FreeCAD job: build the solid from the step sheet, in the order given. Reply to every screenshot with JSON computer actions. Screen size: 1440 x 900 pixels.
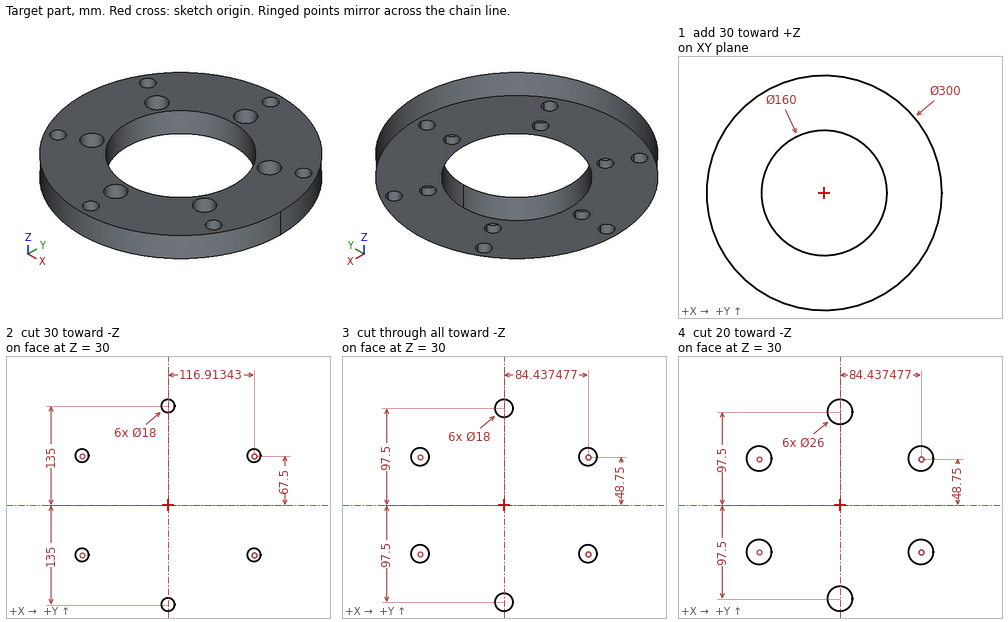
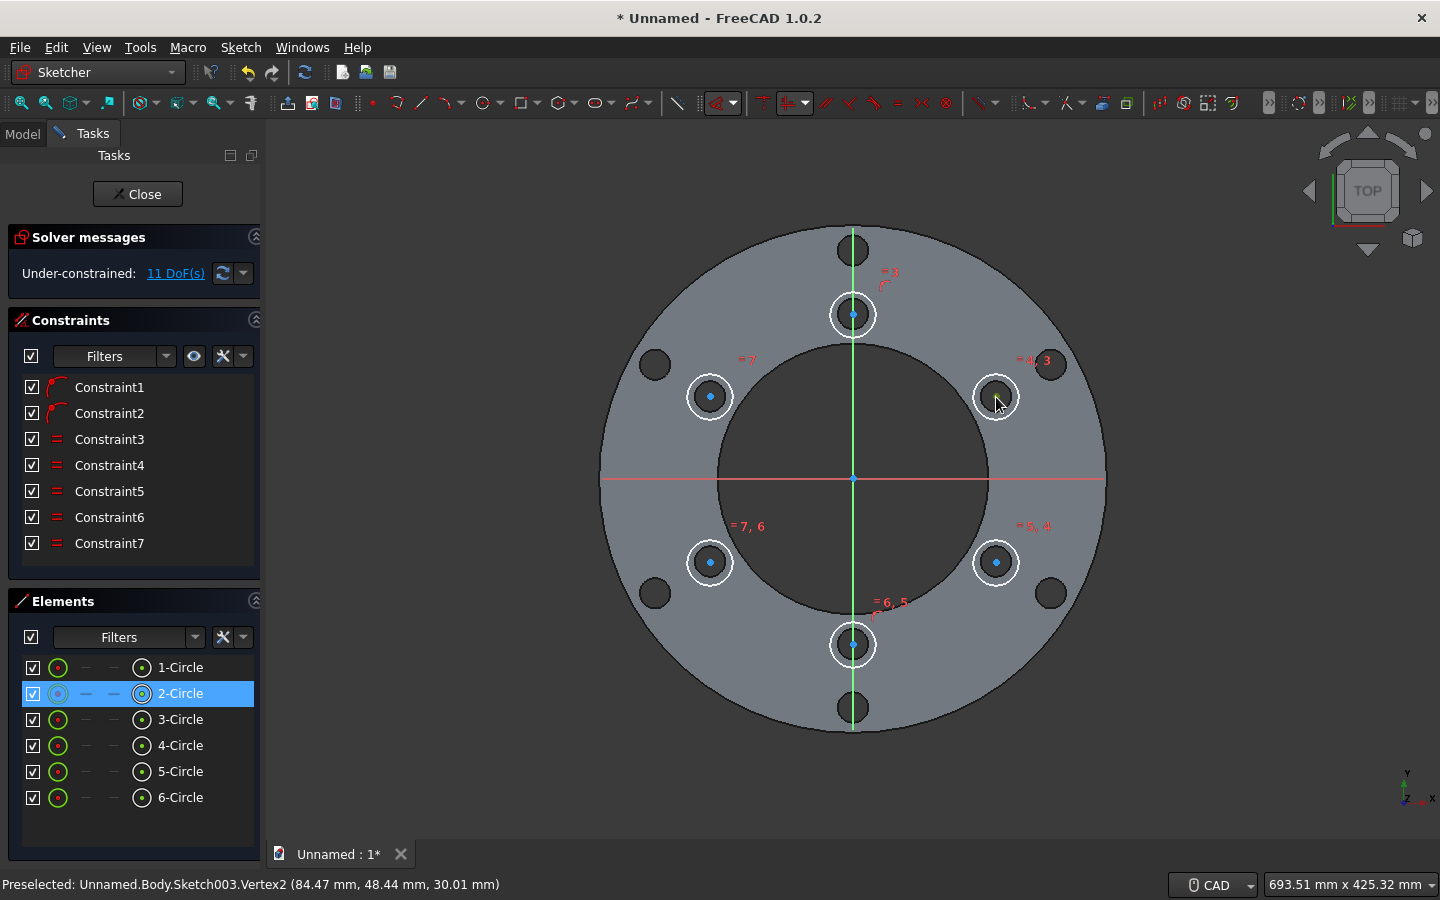
{"action": "left_click", "coordinate": [996, 563]}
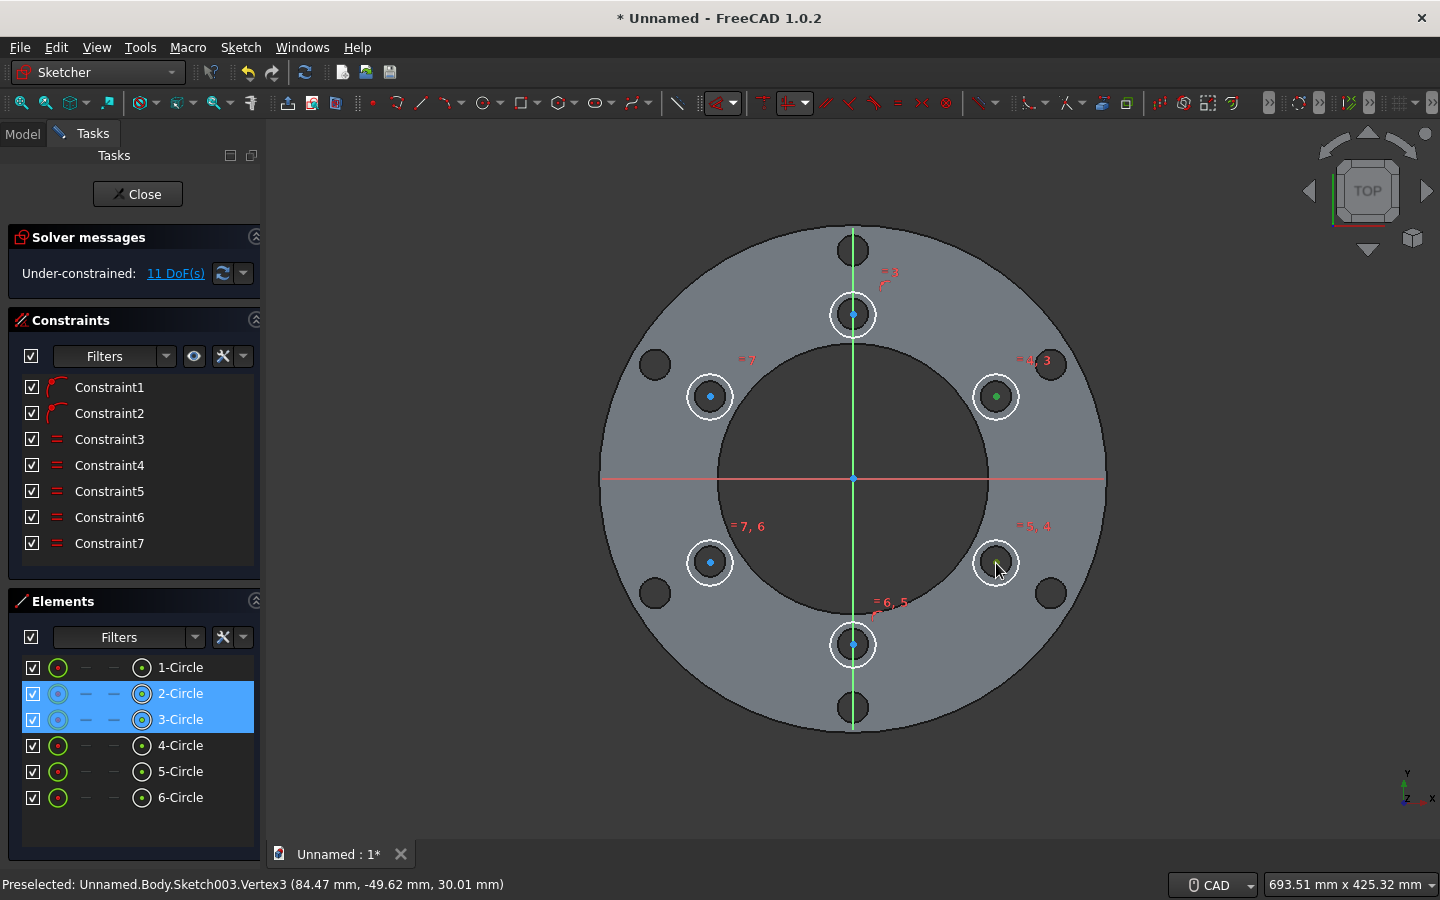
{"action": "left_click", "coordinate": [644, 479]}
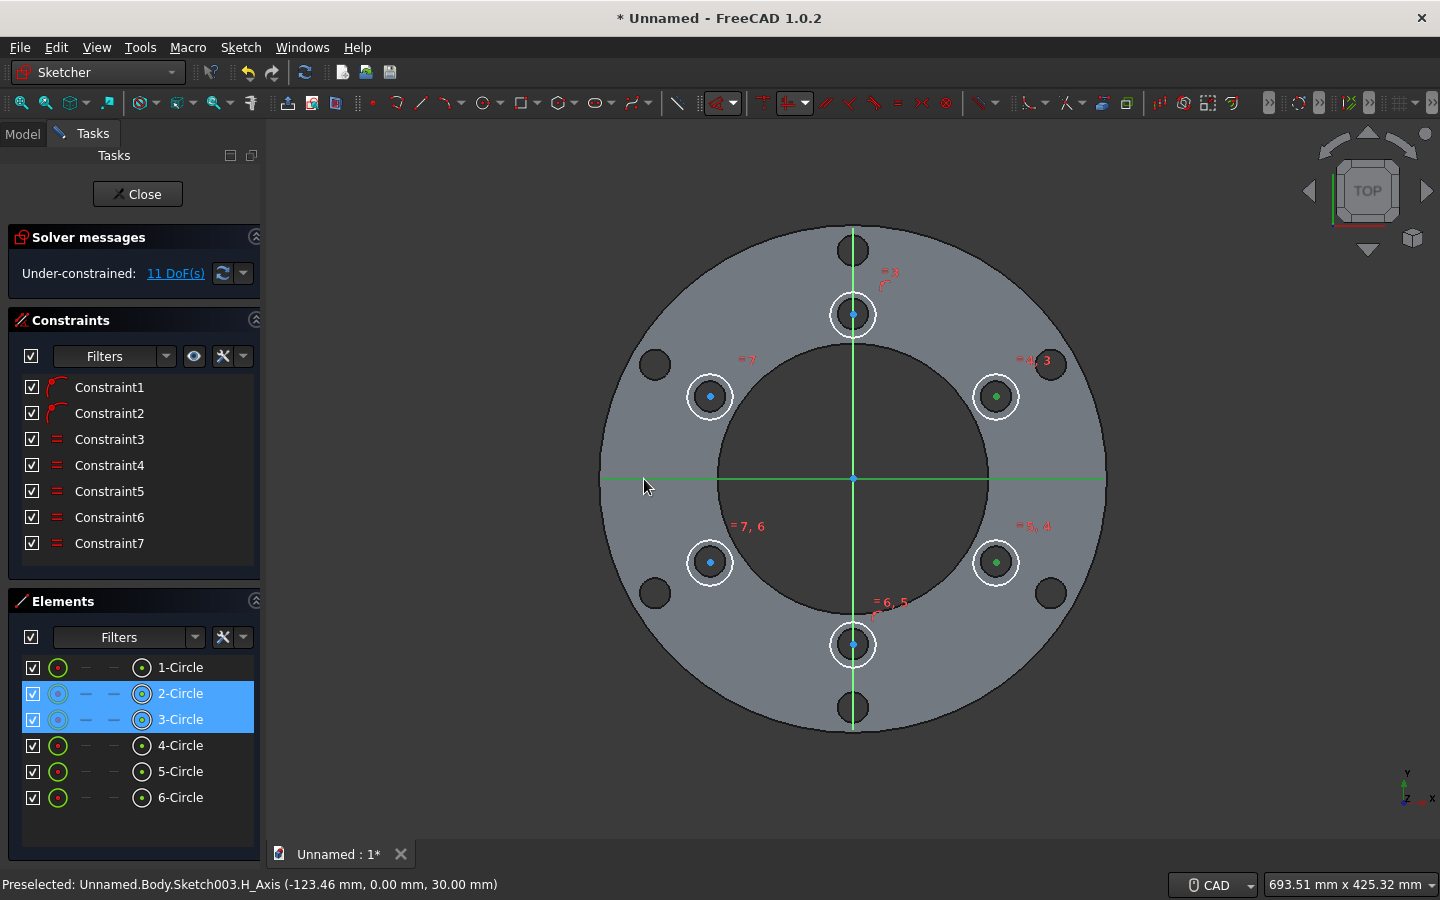
{"action": "left_click", "coordinate": [922, 104]}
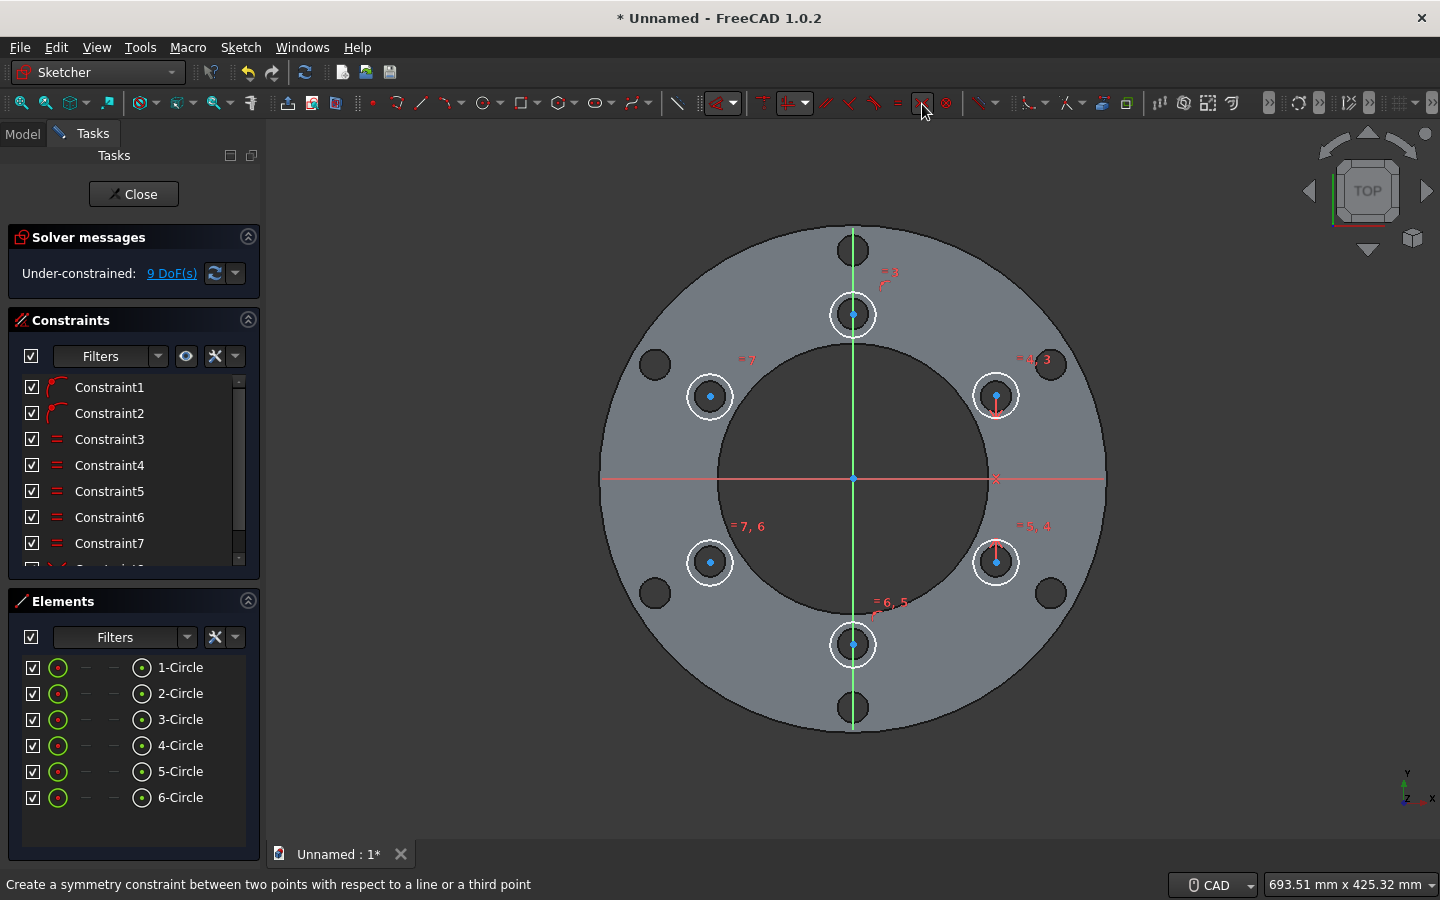
{"action": "left_click", "coordinate": [996, 563]}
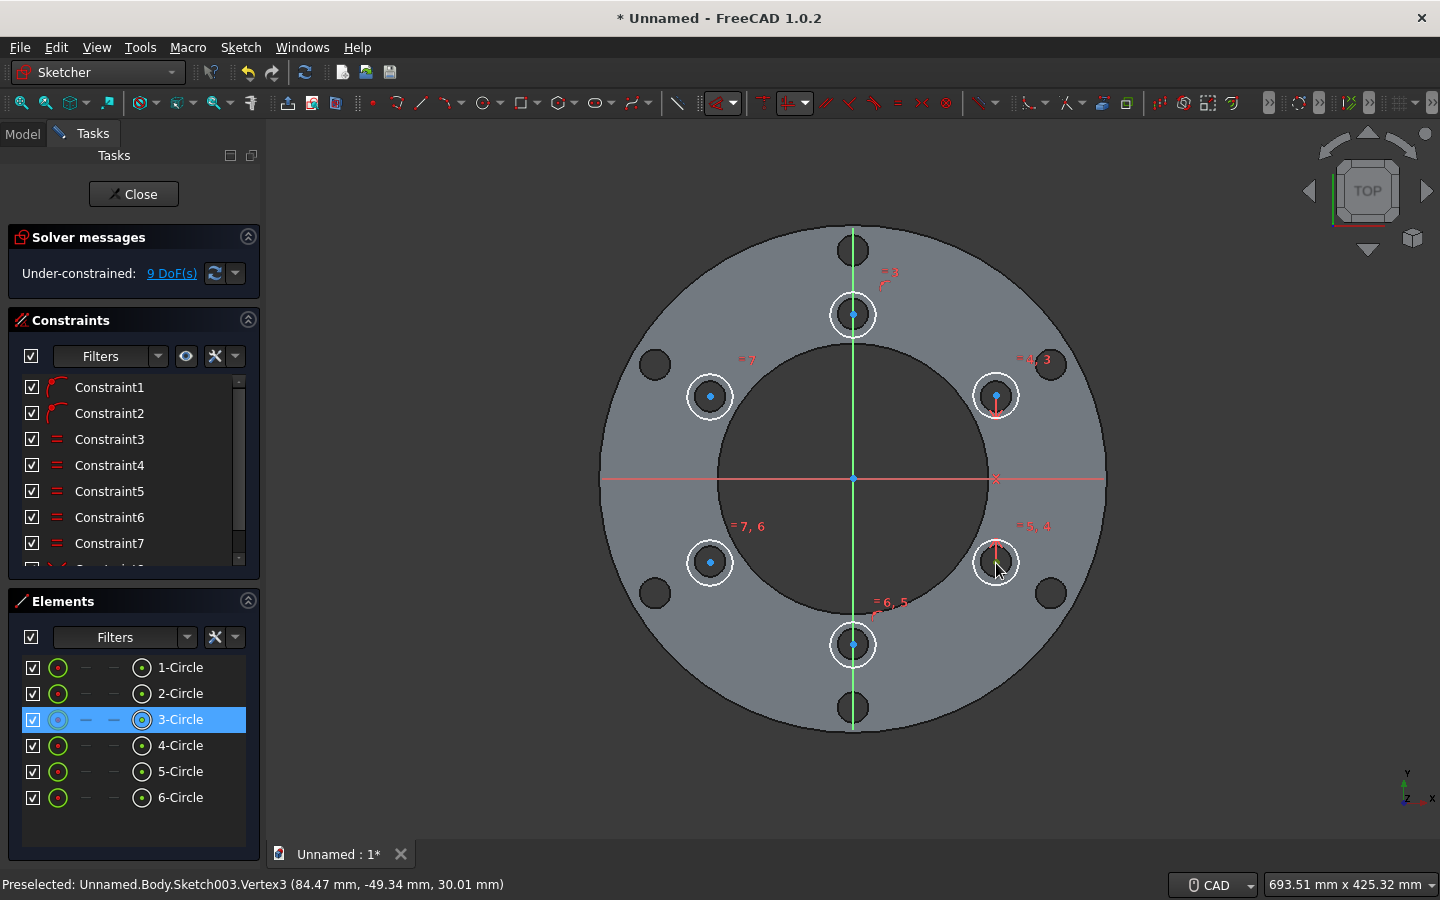
{"action": "left_click", "coordinate": [710, 563]}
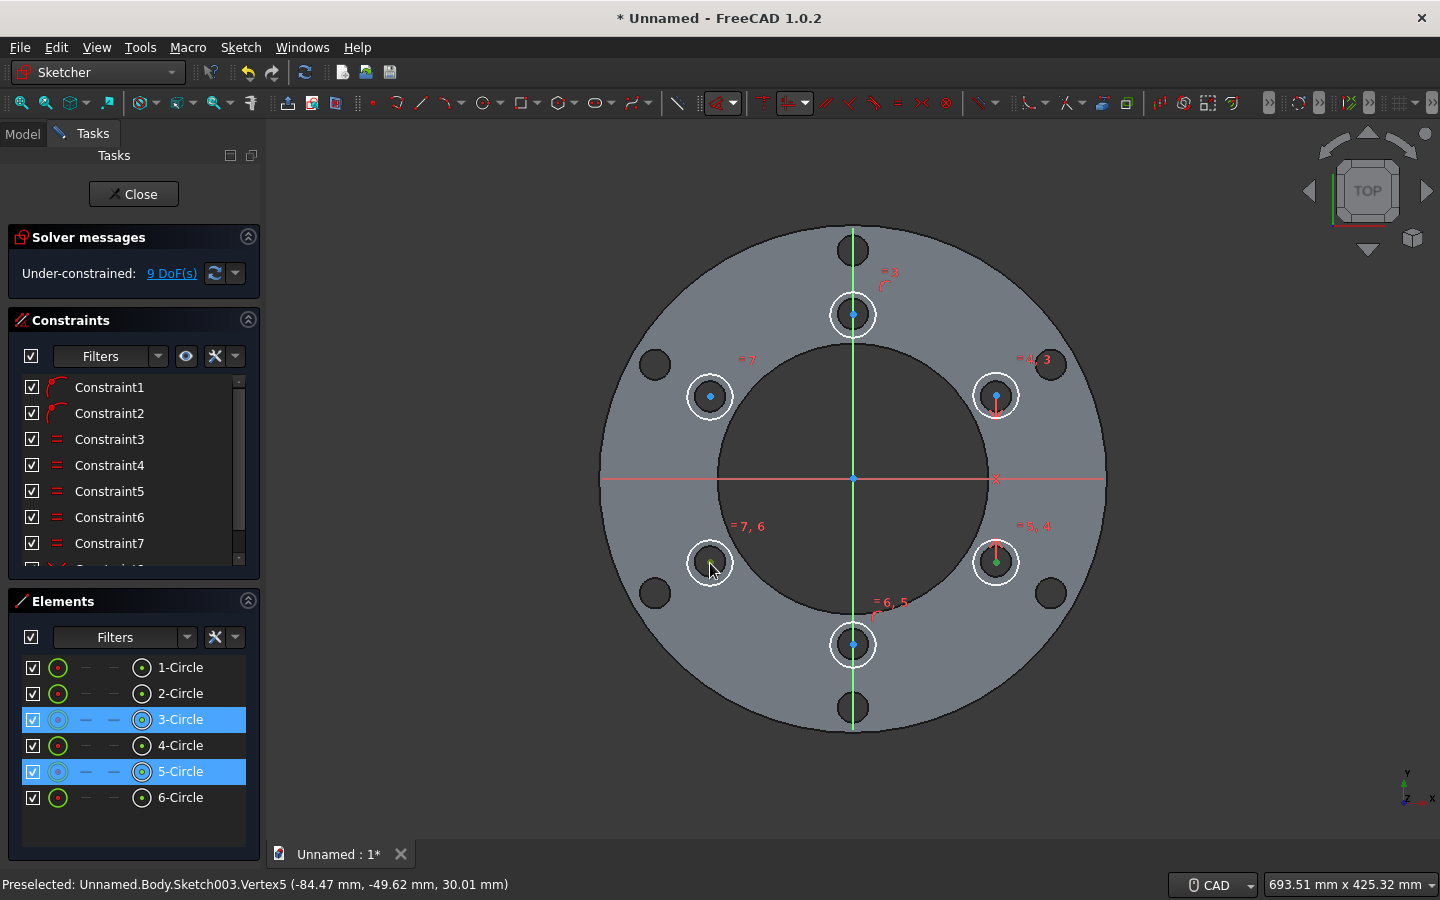
{"action": "left_click", "coordinate": [853, 716]}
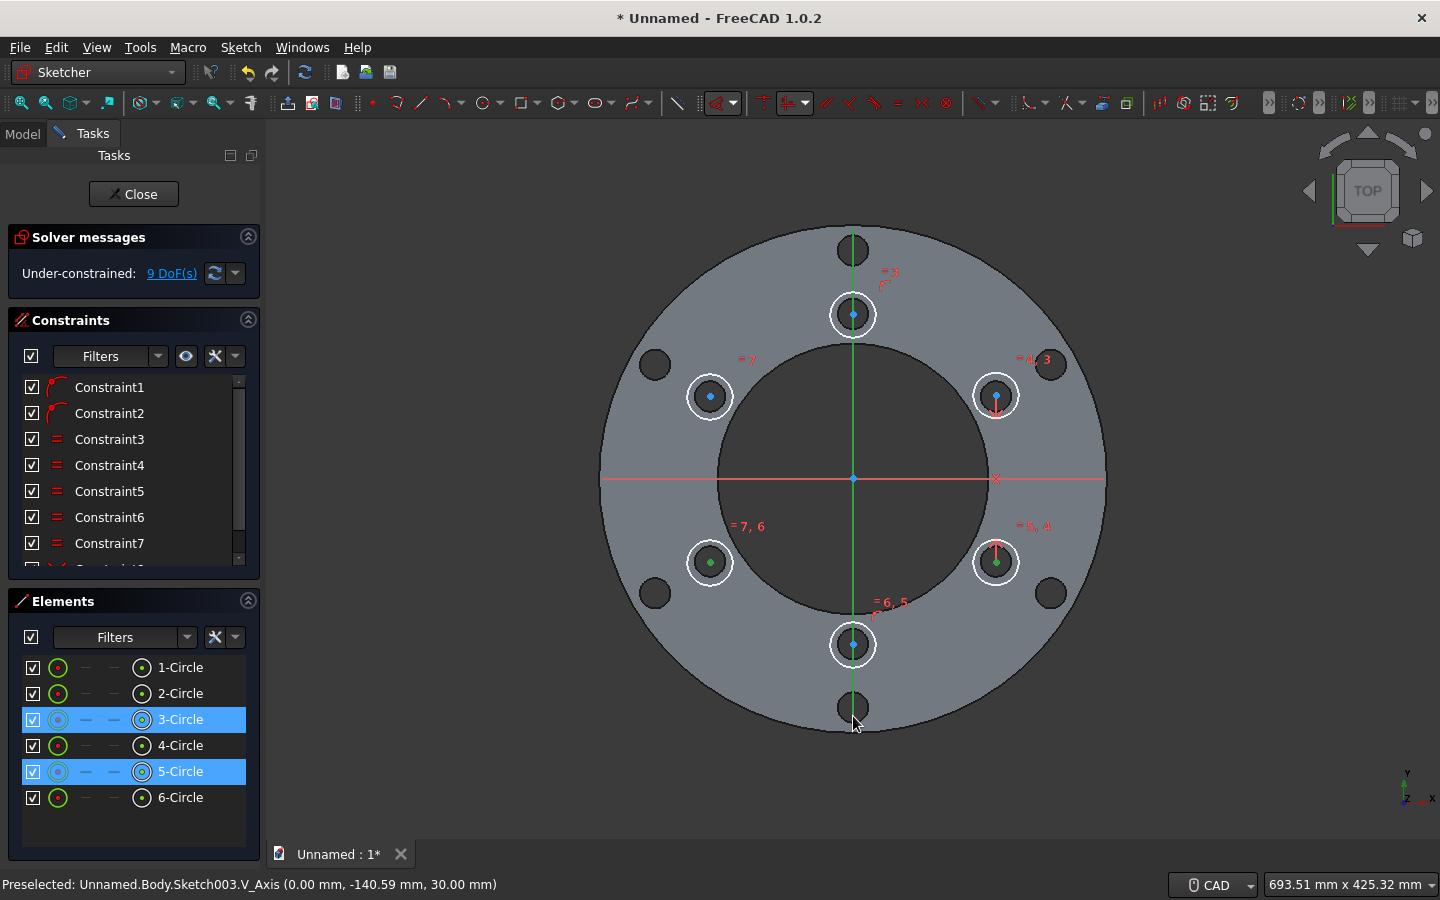
{"action": "key", "text": "s"}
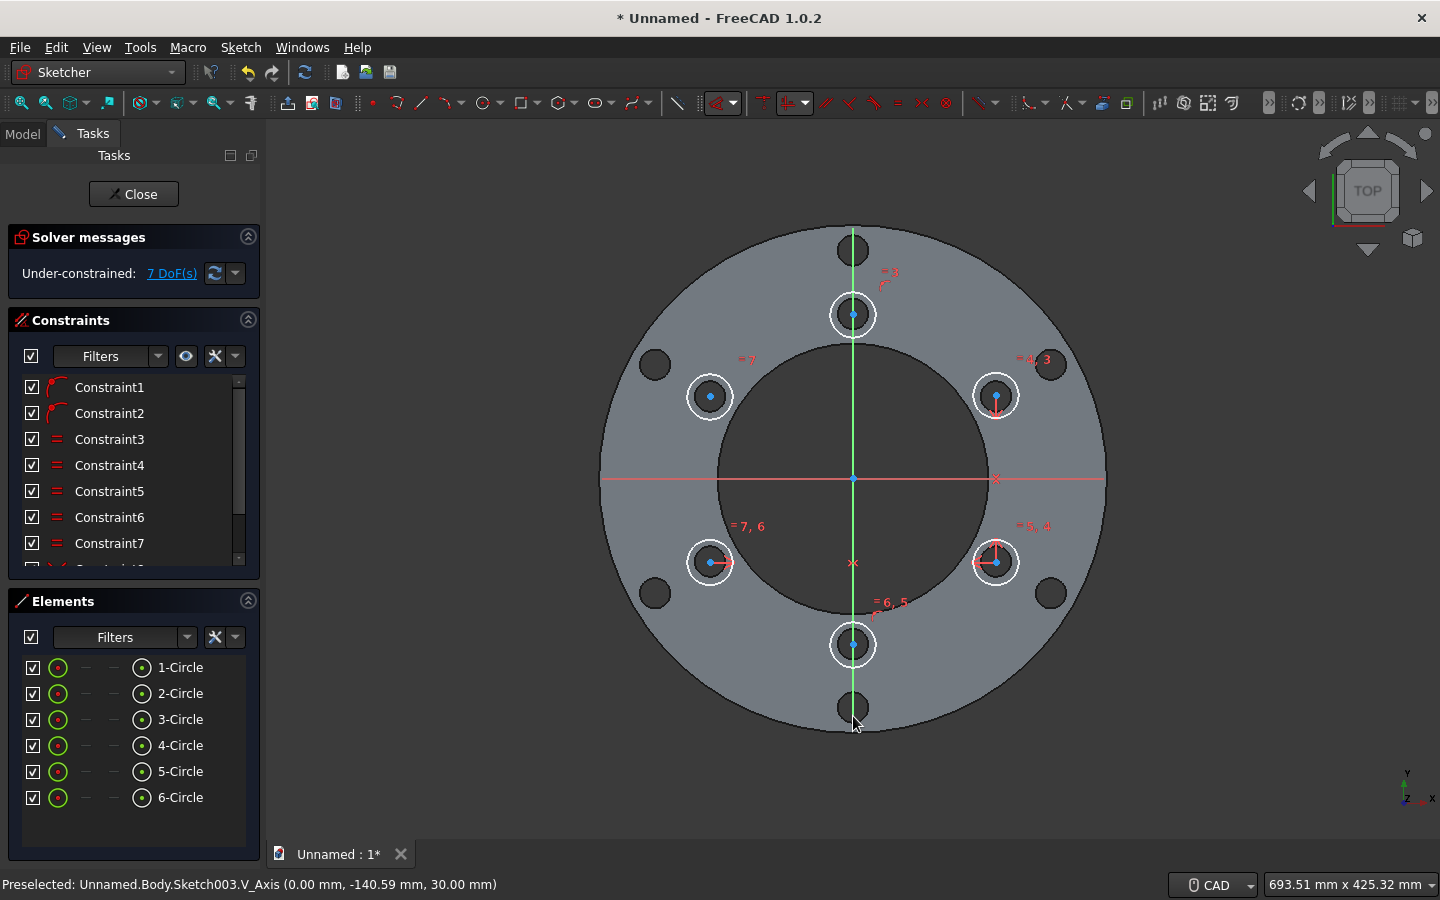
{"action": "left_click", "coordinate": [996, 395]}